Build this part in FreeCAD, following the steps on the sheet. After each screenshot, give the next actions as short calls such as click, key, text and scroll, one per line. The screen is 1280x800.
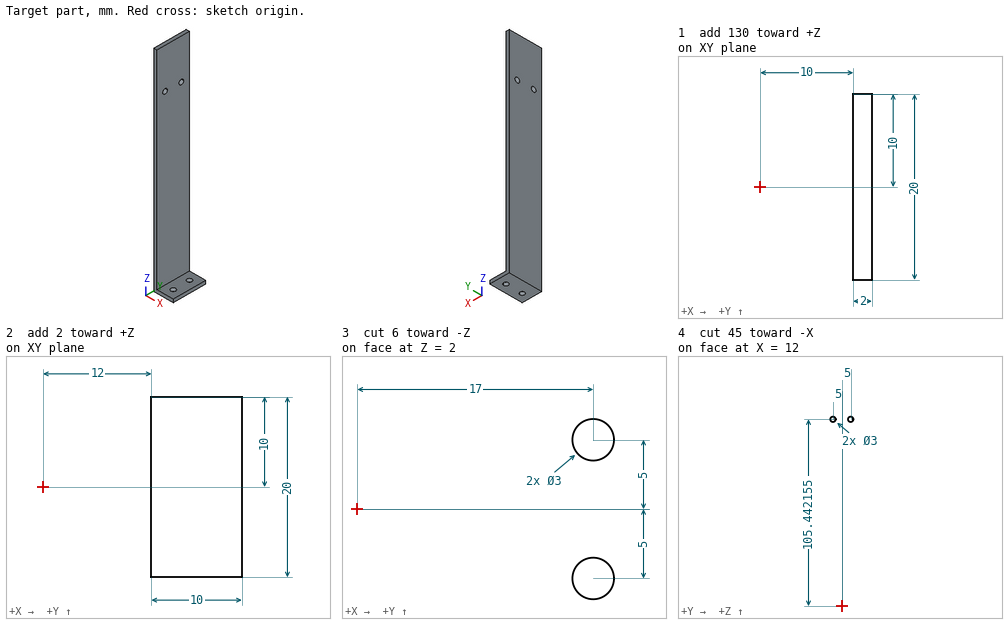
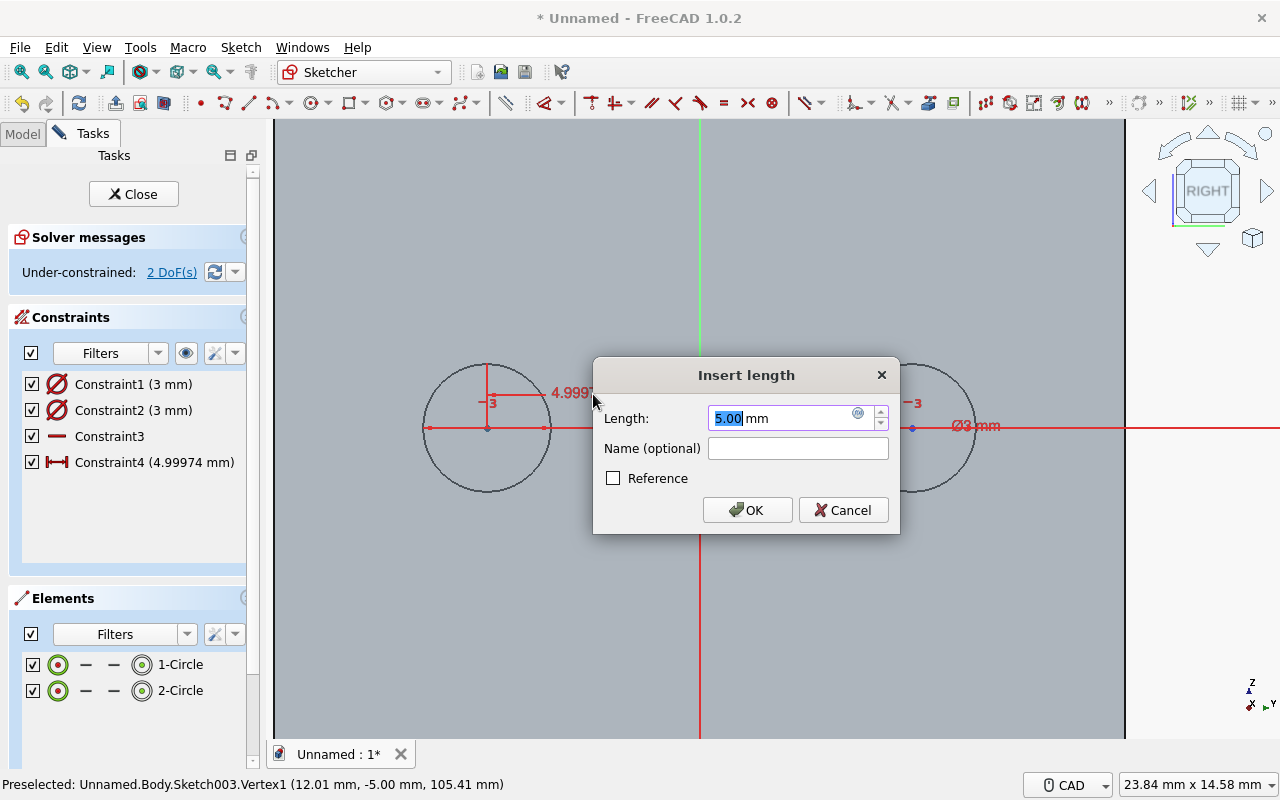
text(5)
key(Return)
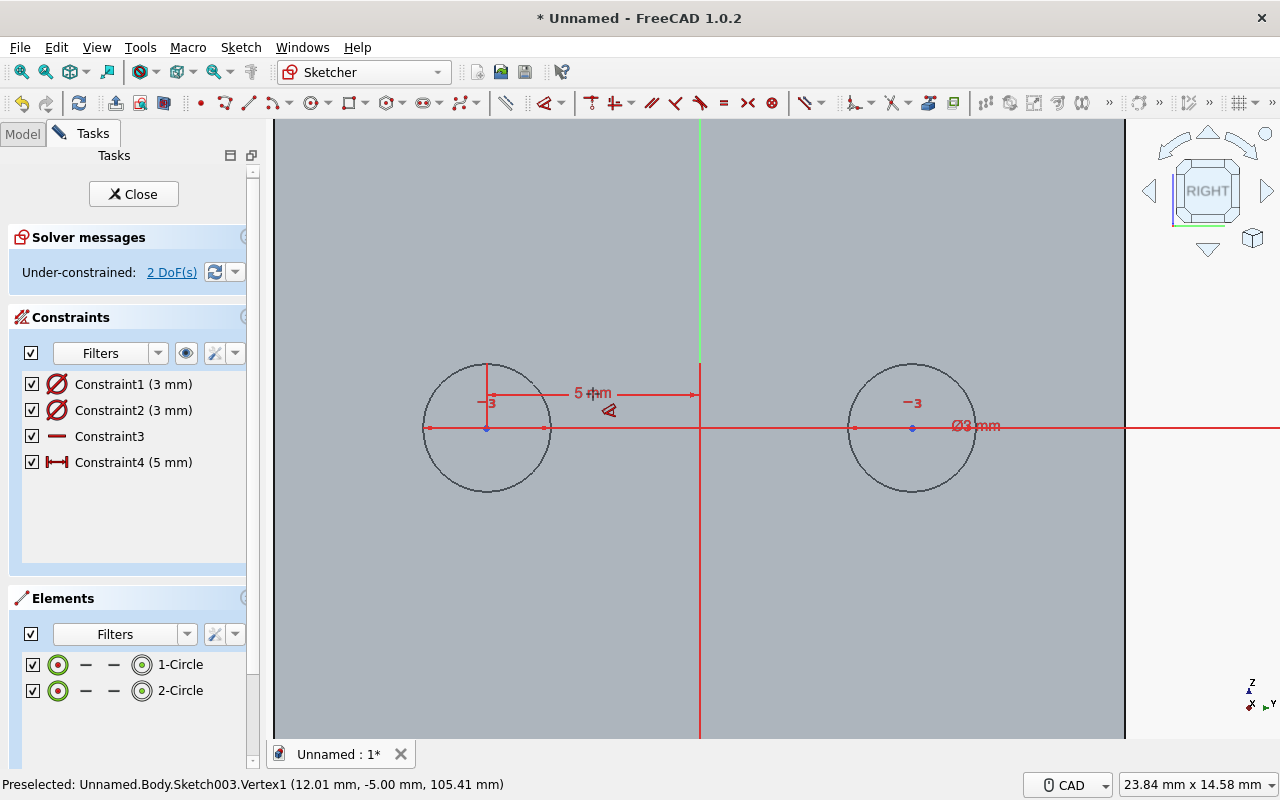
click(912, 428)
click(806, 394)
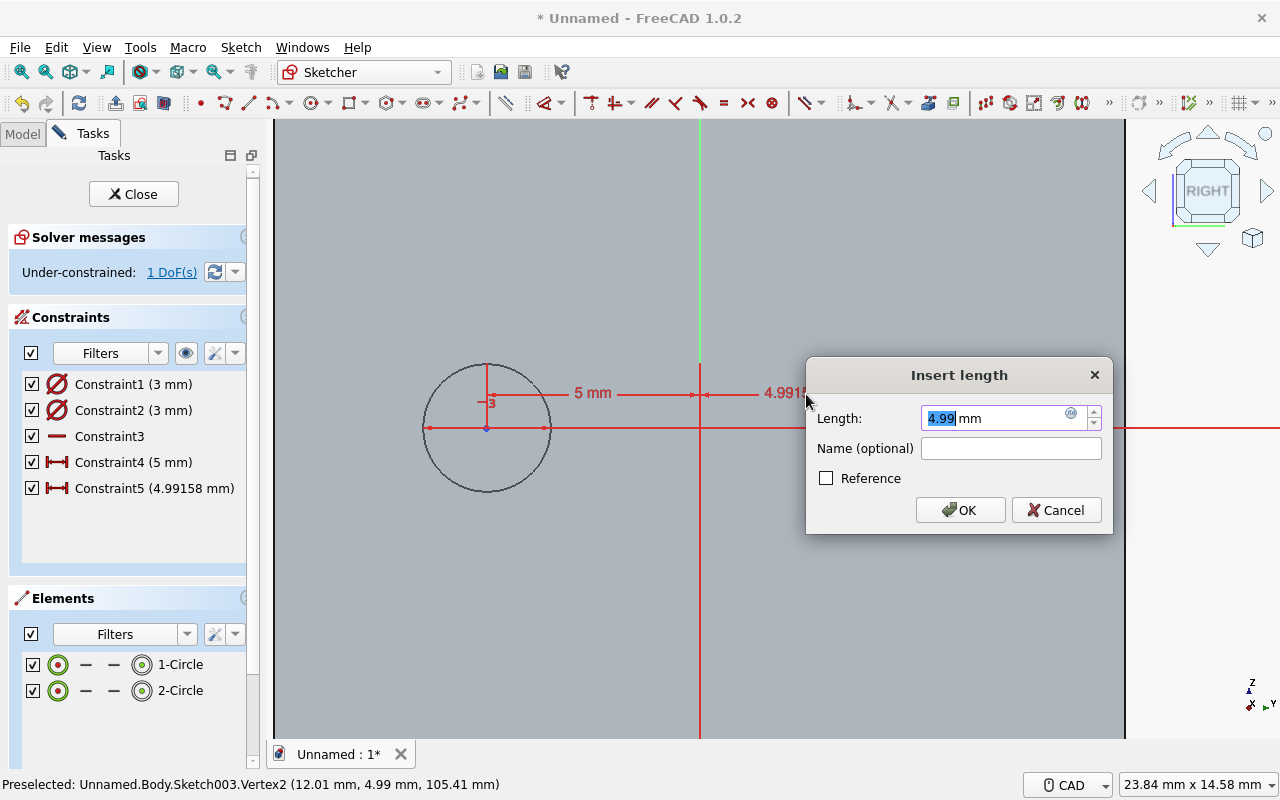
text(5)
key(Return)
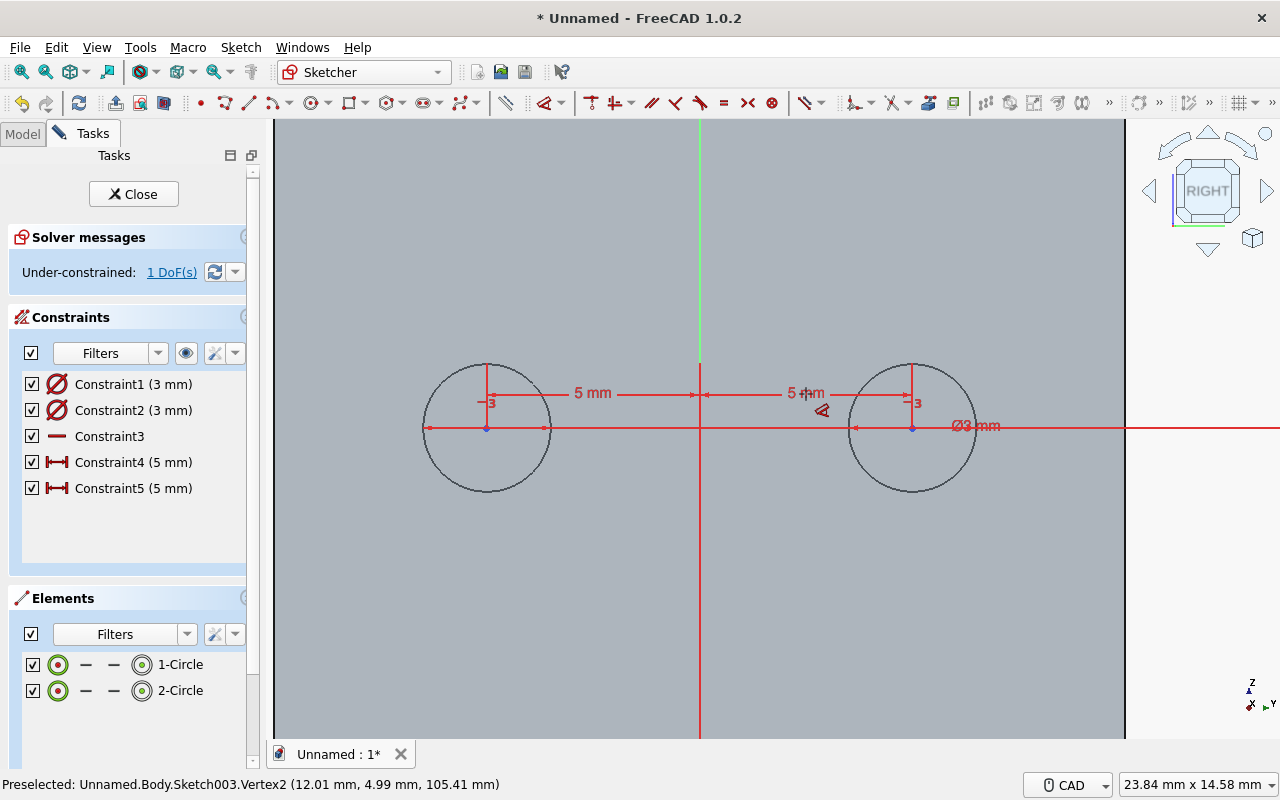
click(487, 428)
click(453, 570)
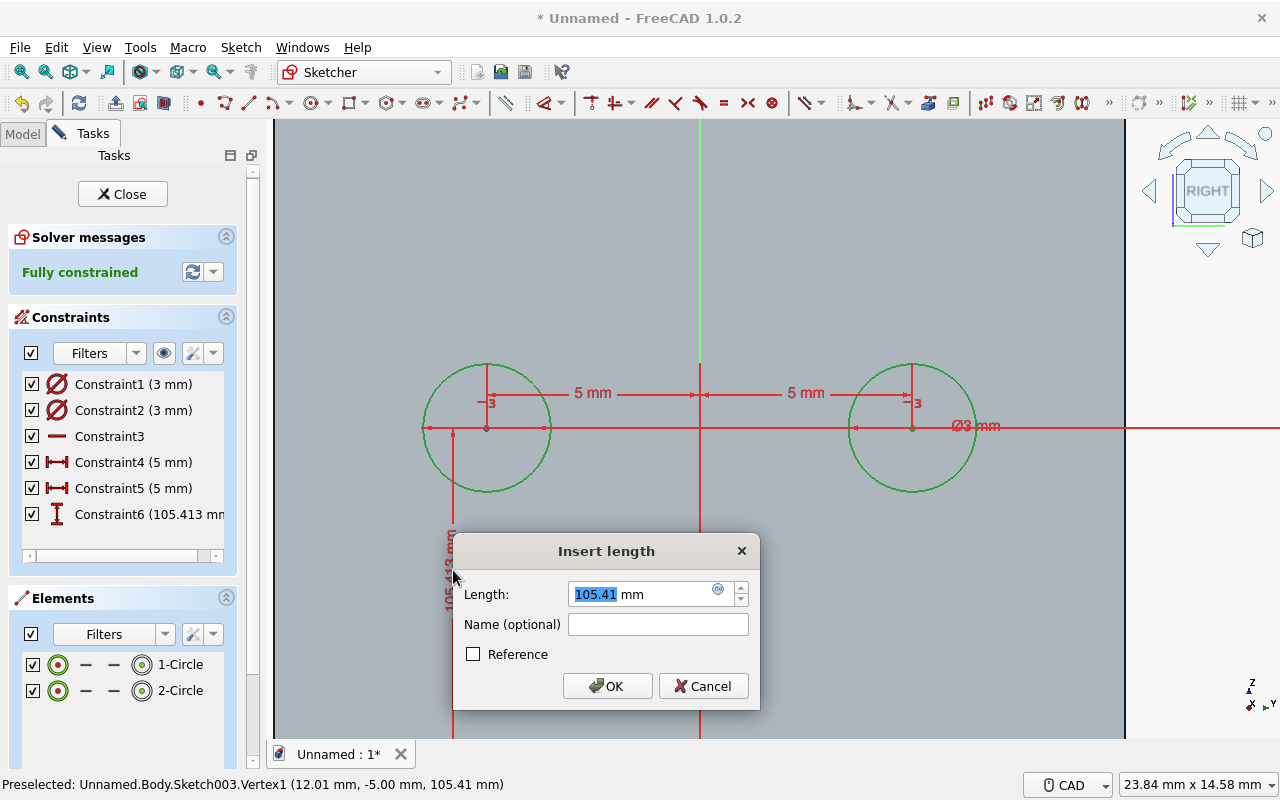
text(105.442155)
key(Return)
key(Escape)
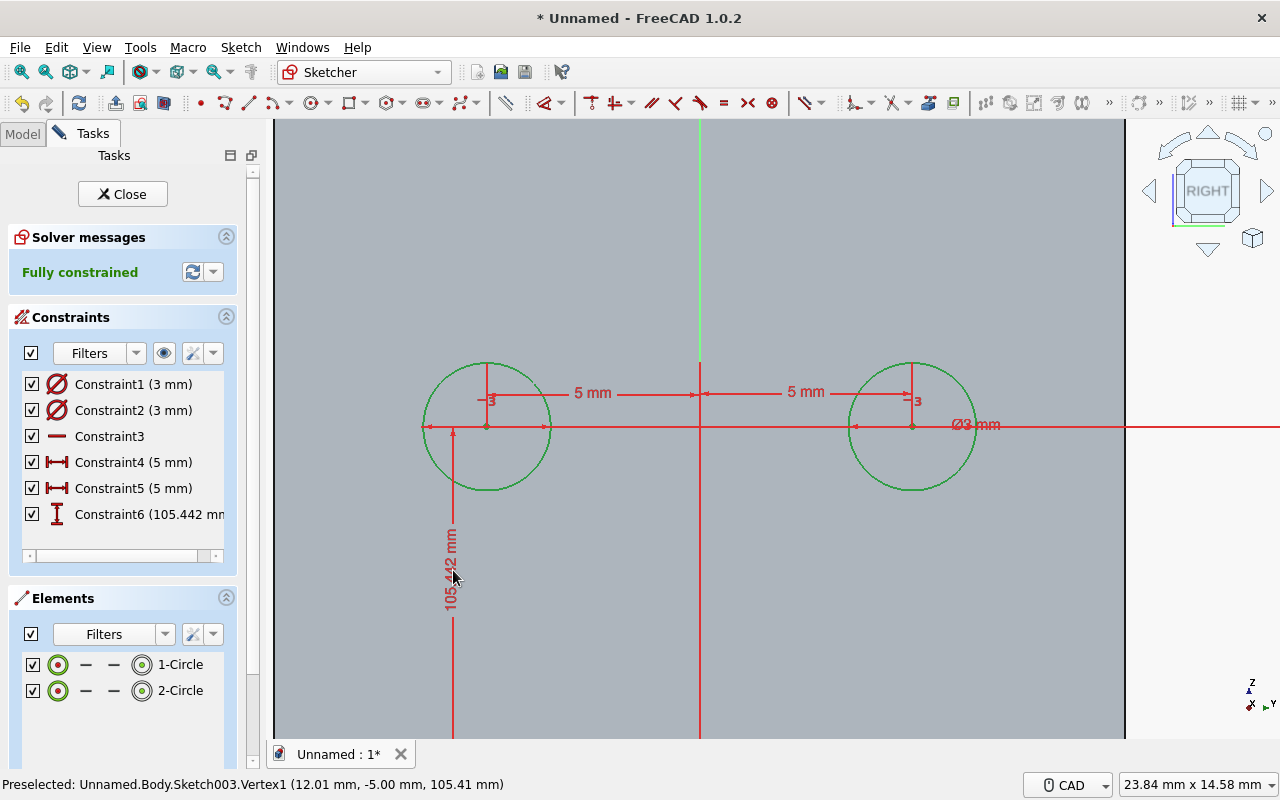
click(123, 194)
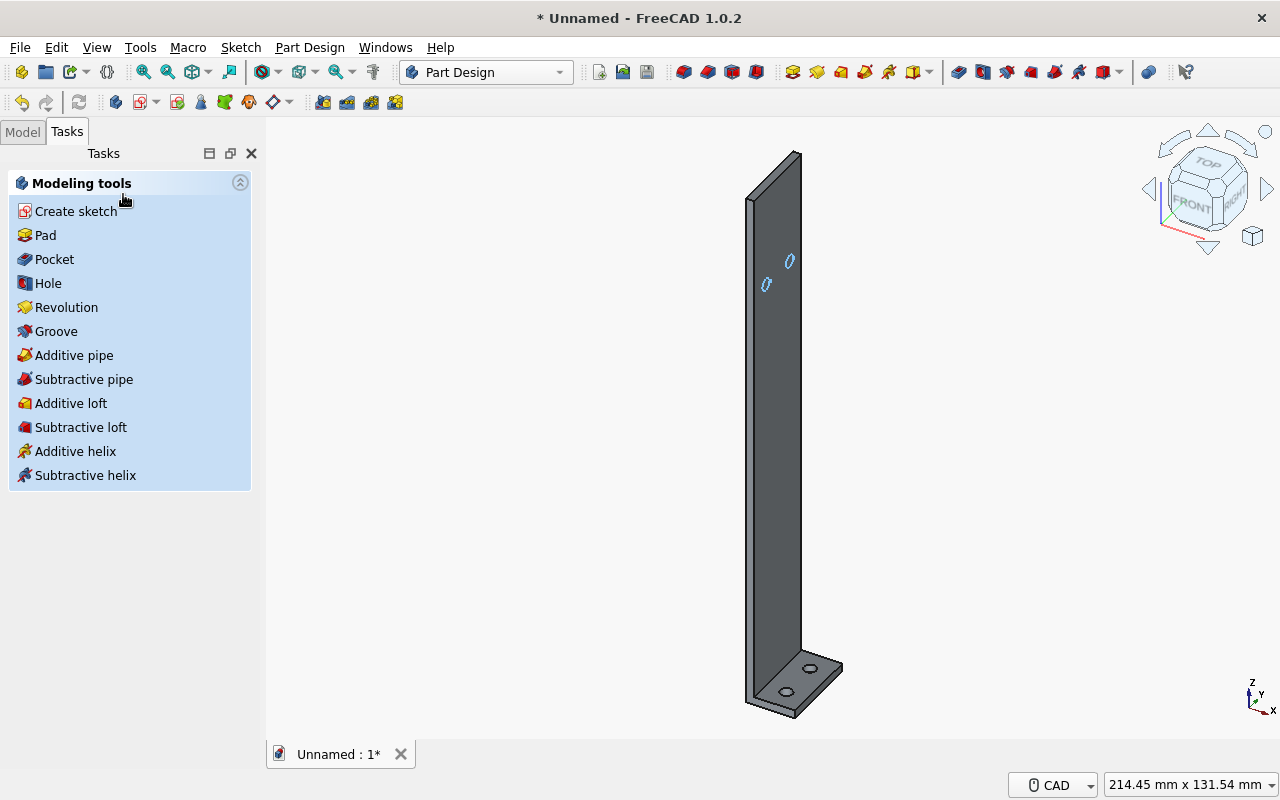
click(960, 72)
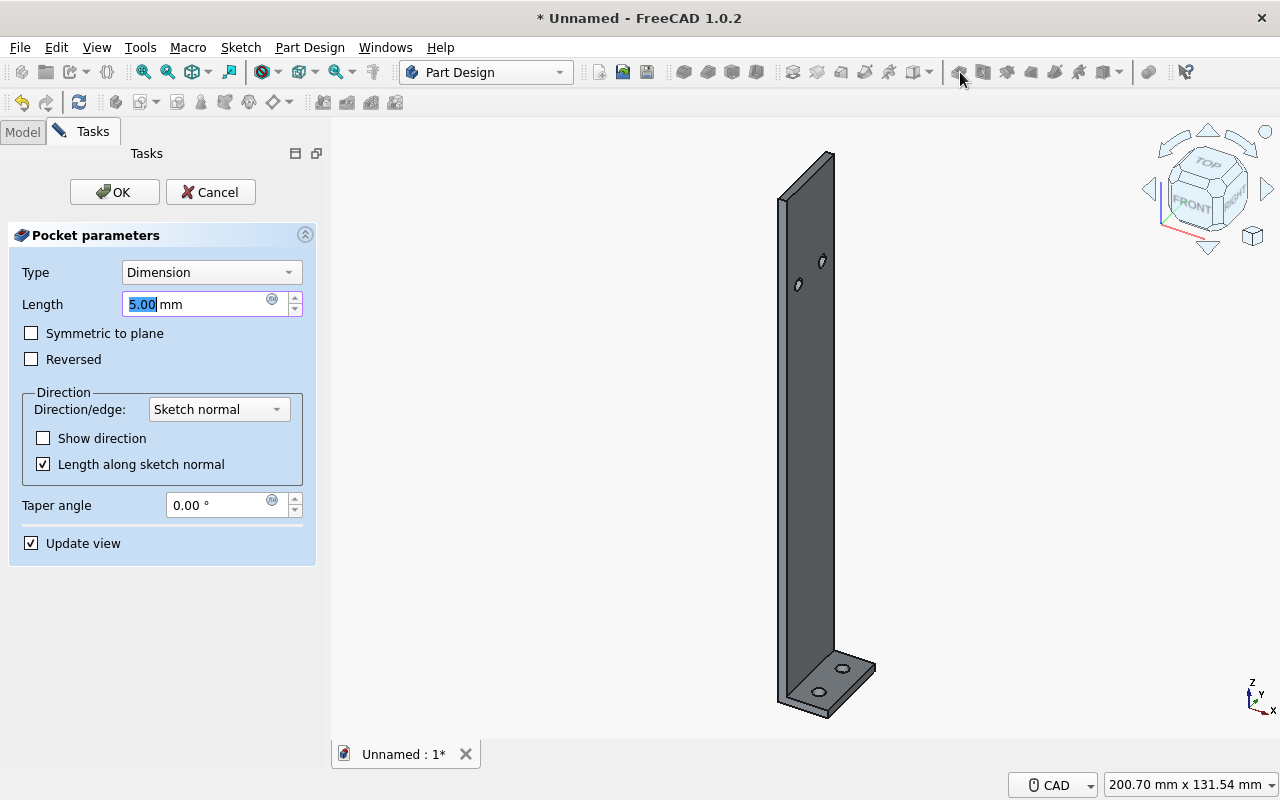
text(45)
key(Tab)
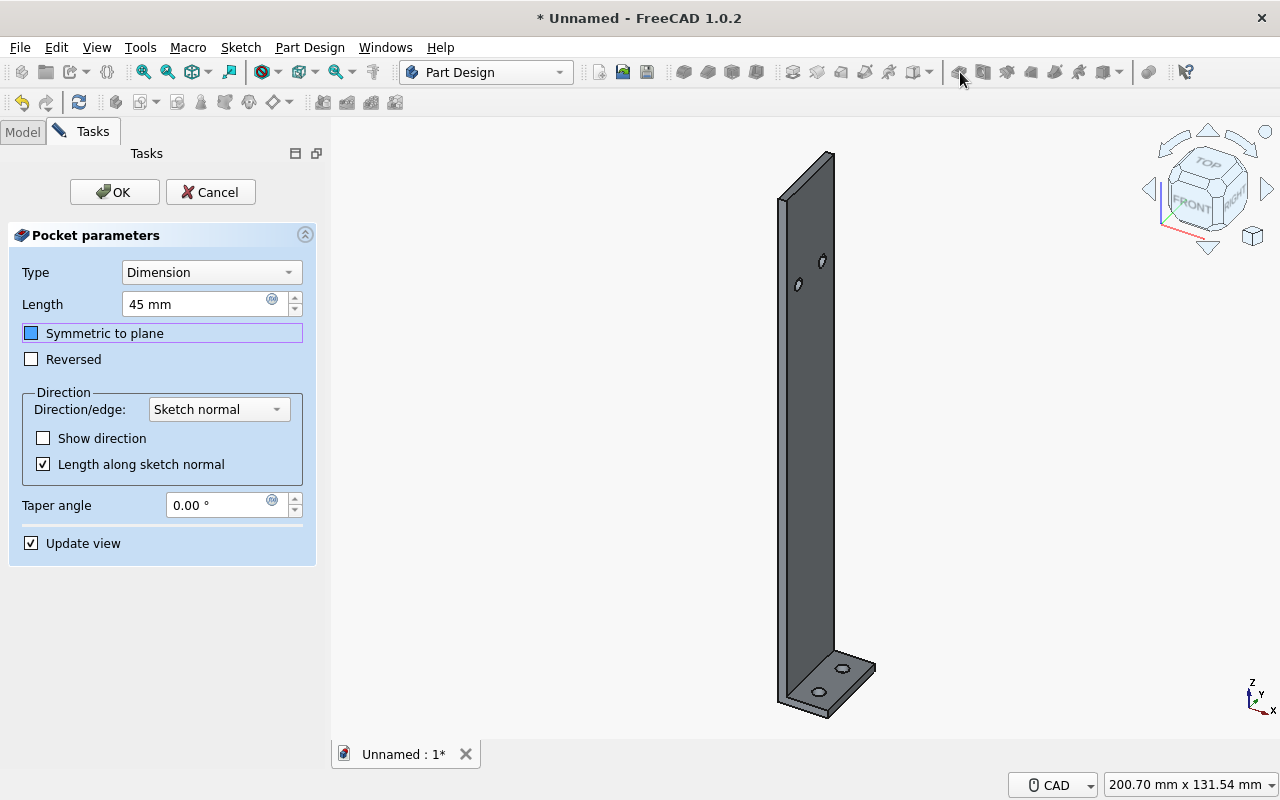
click(115, 192)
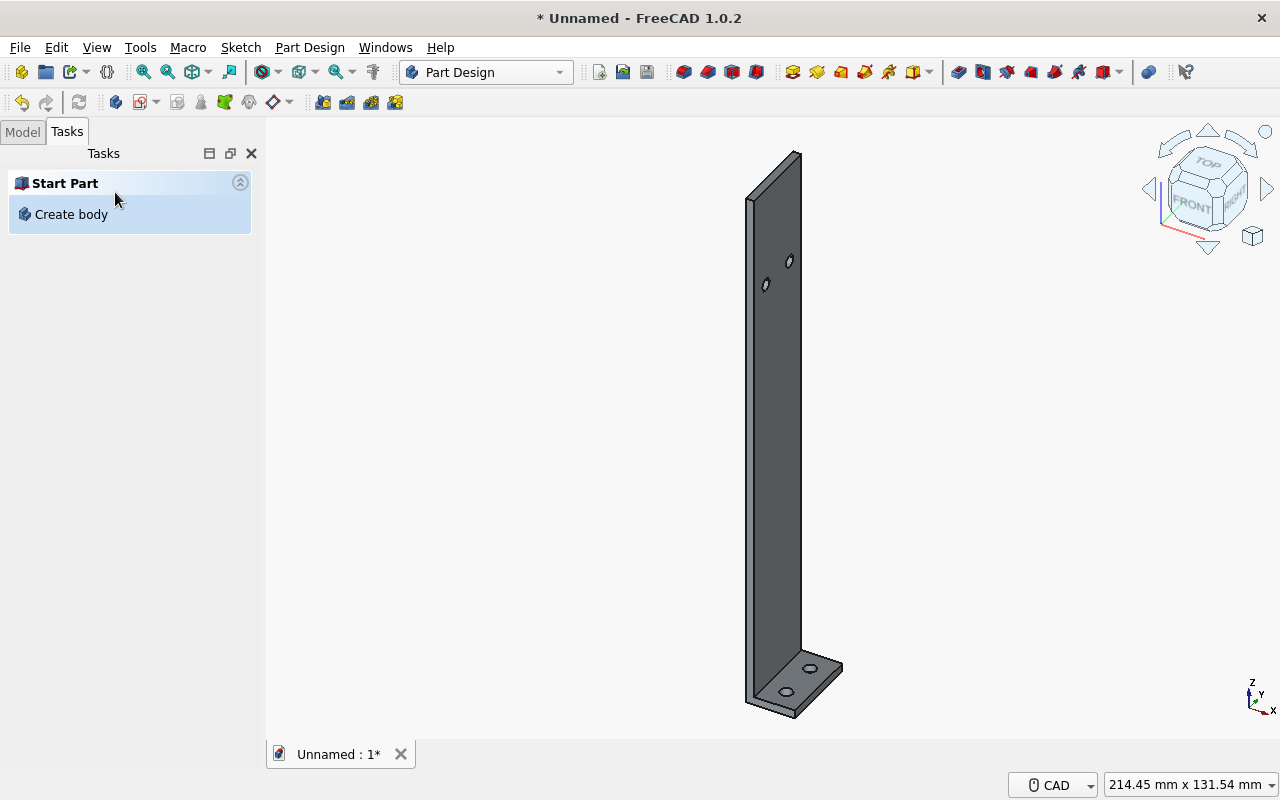
key(0)